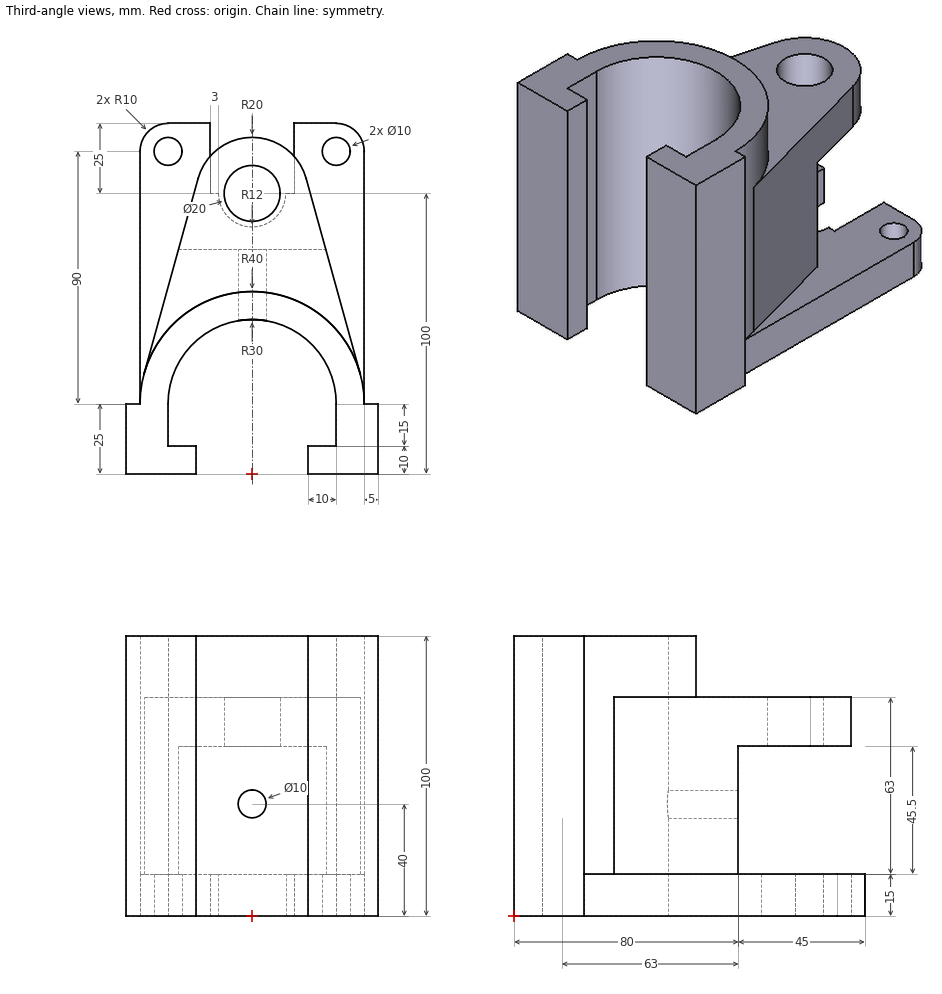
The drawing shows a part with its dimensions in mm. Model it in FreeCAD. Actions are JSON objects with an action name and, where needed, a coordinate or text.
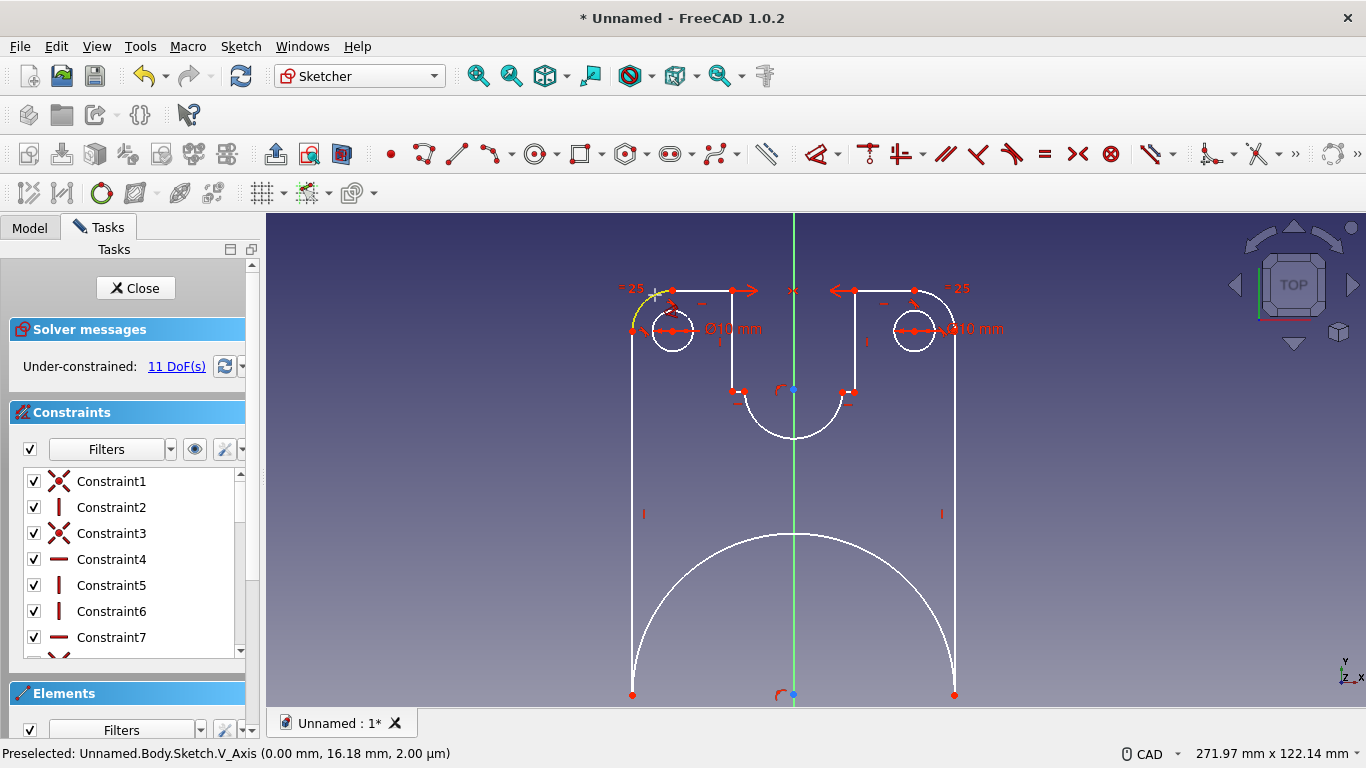
{"action": "left_click", "coordinate": [654, 295]}
{"action": "left_click", "coordinate": [639, 267]}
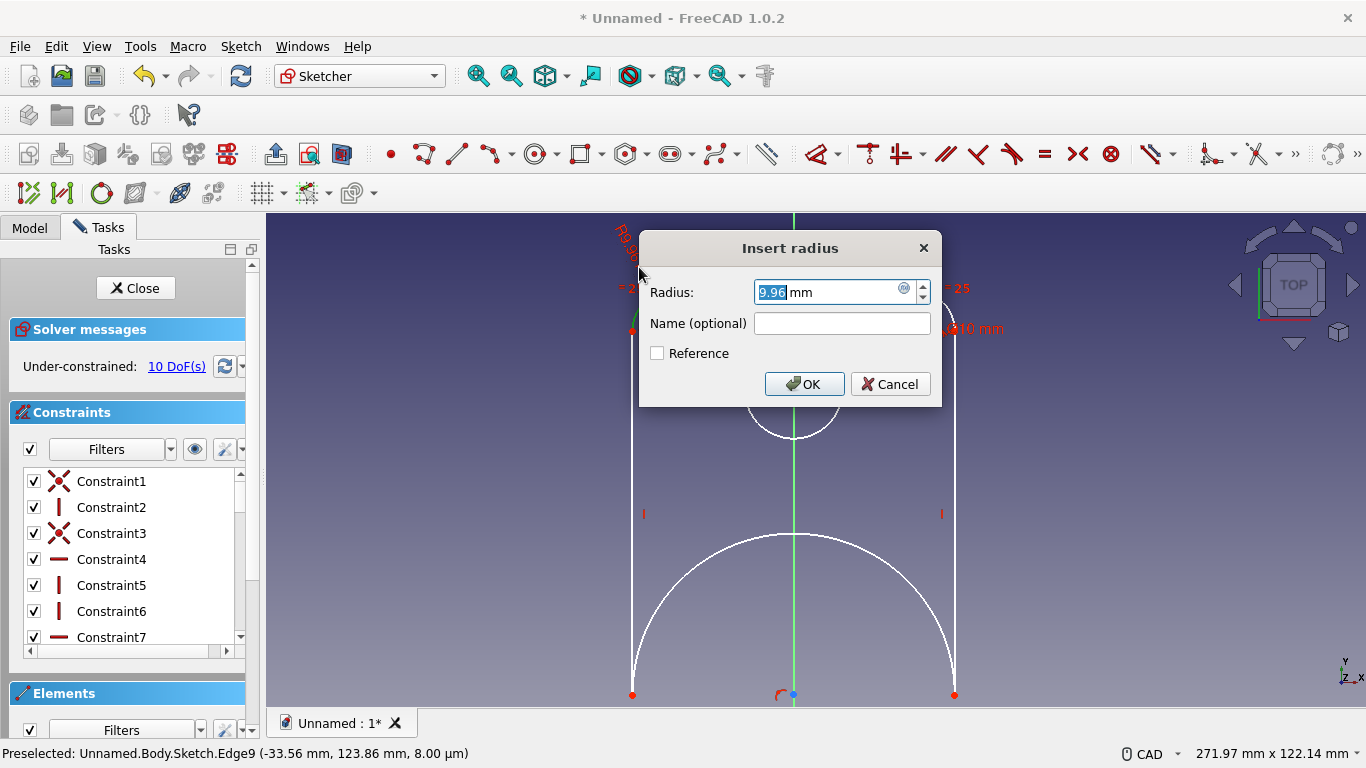
{"action": "type", "text": "10"}
{"action": "key", "text": "Return"}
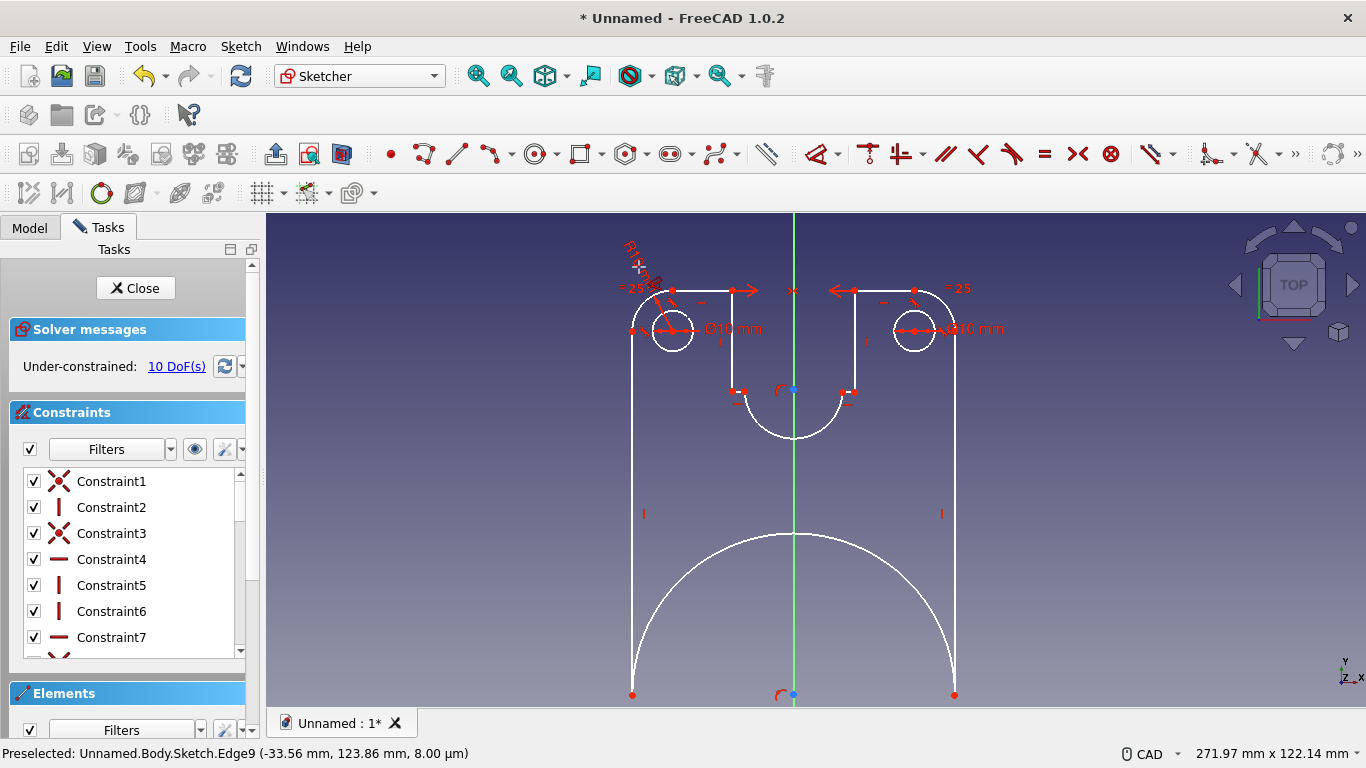
{"action": "left_click", "coordinate": [889, 564]}
{"action": "left_click", "coordinate": [908, 538]}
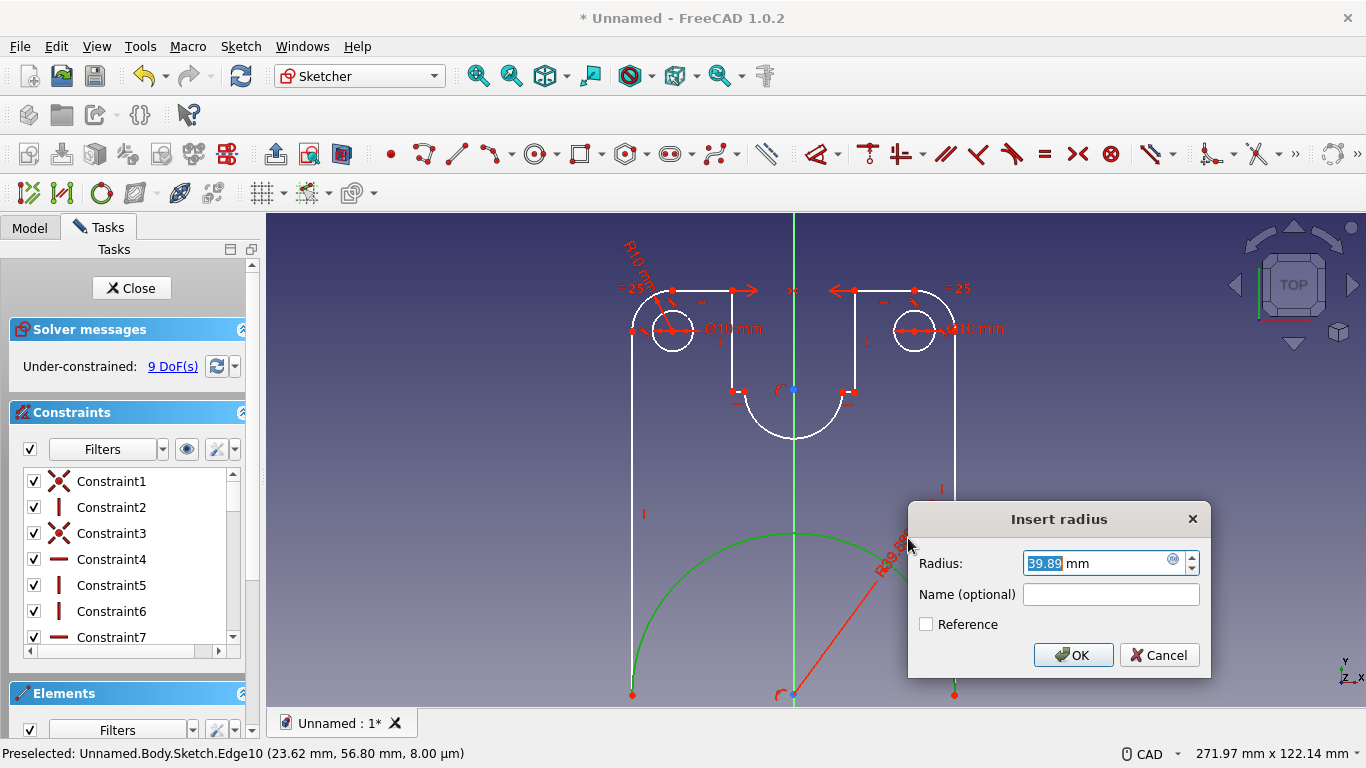
{"action": "type", "text": "40"}
{"action": "key", "text": "Return"}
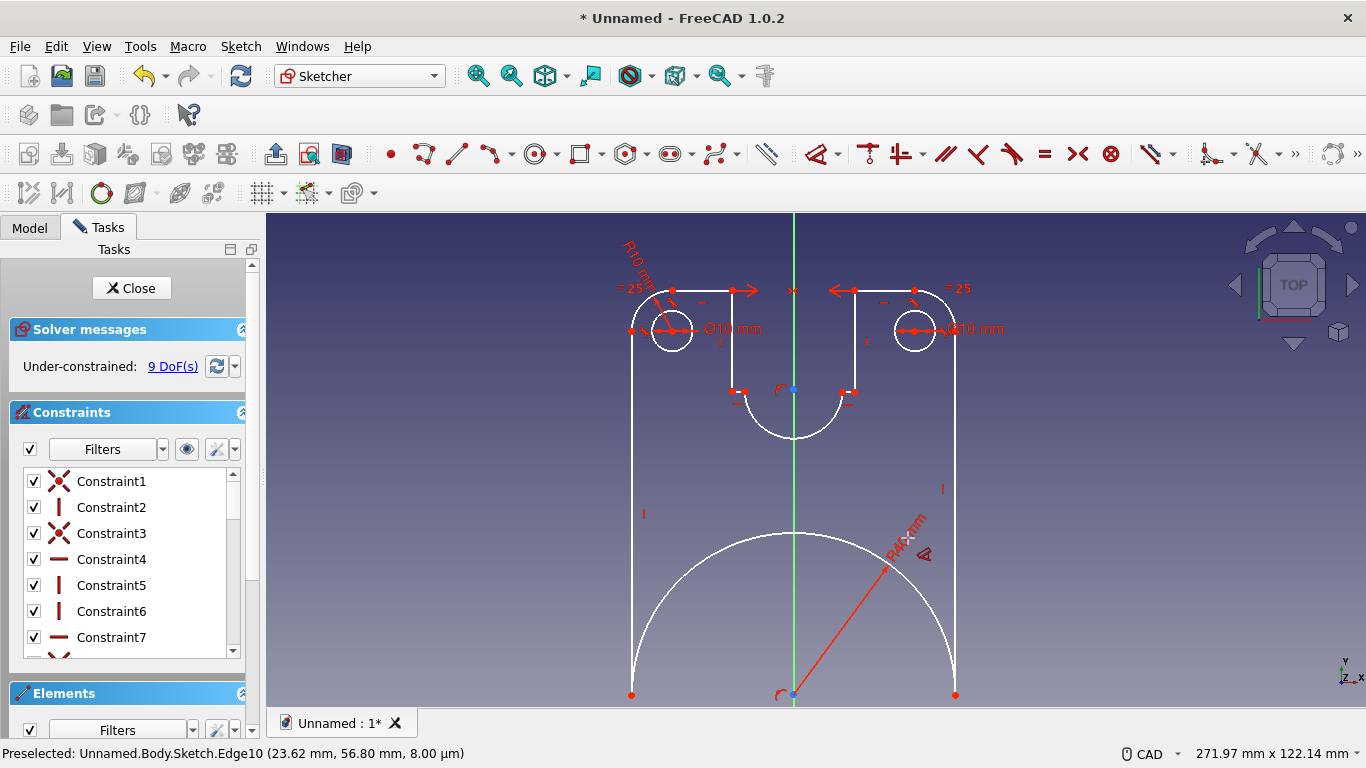
{"action": "left_click", "coordinate": [765, 430]}
{"action": "left_click", "coordinate": [746, 456]}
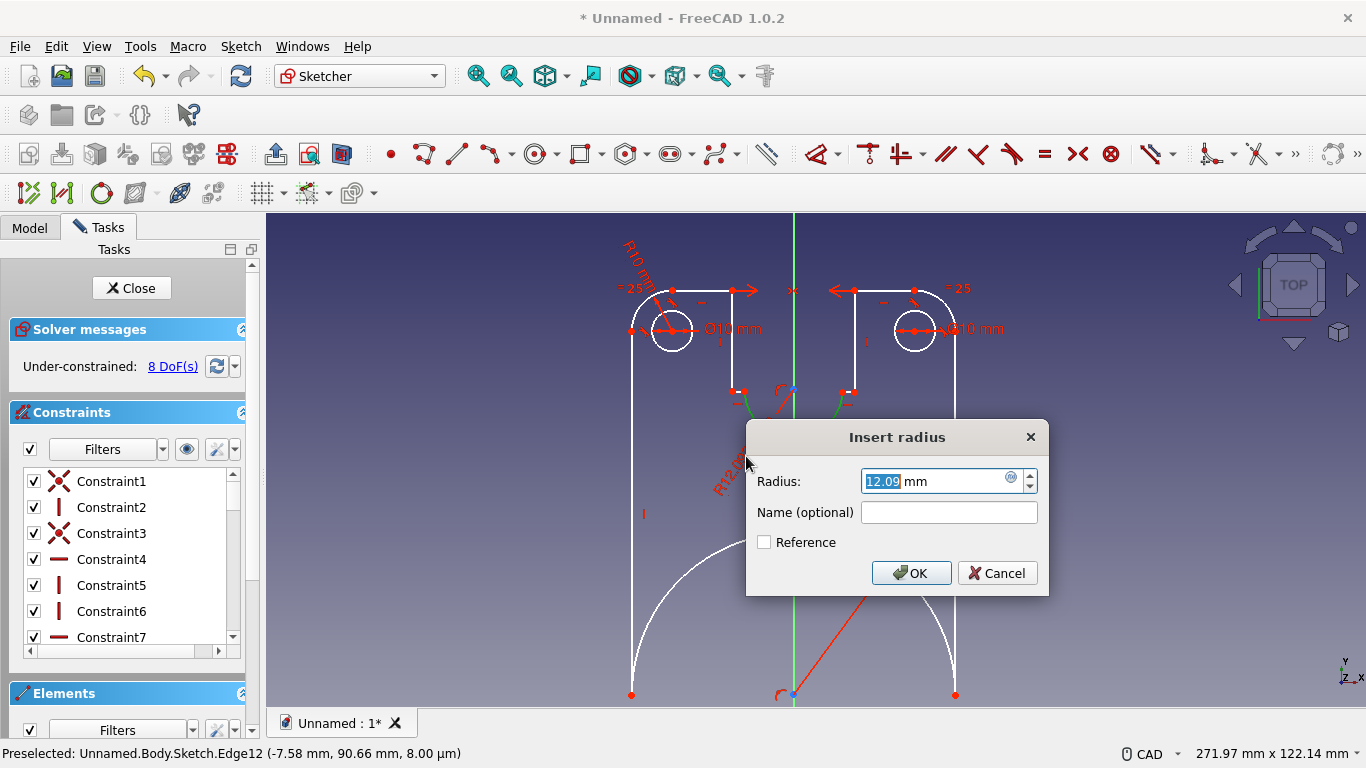
{"action": "type", "text": "12"}
{"action": "key", "text": "Return"}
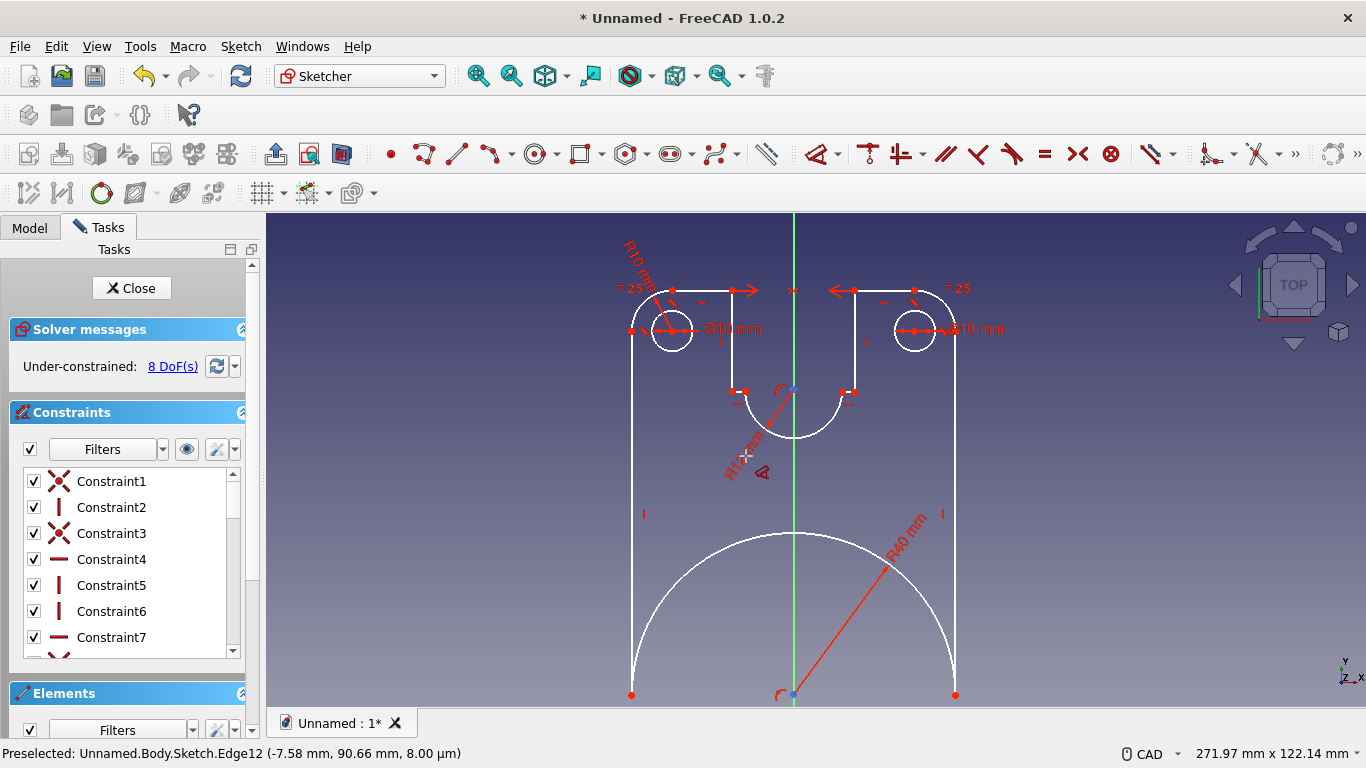
{"action": "scroll", "coordinate": [739, 392], "scroll_direction": "up", "scroll_amount": 6}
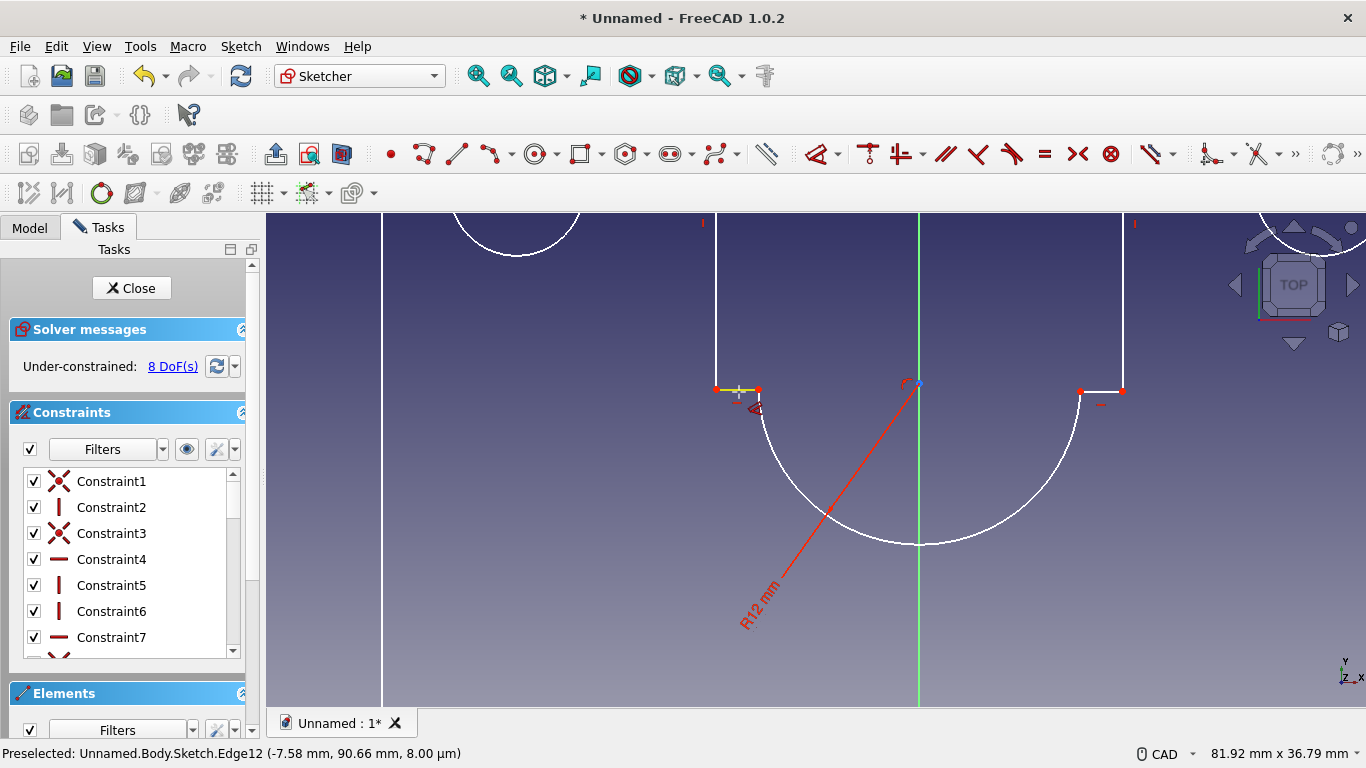
{"action": "left_click", "coordinate": [737, 390]}
{"action": "left_click", "coordinate": [737, 356]}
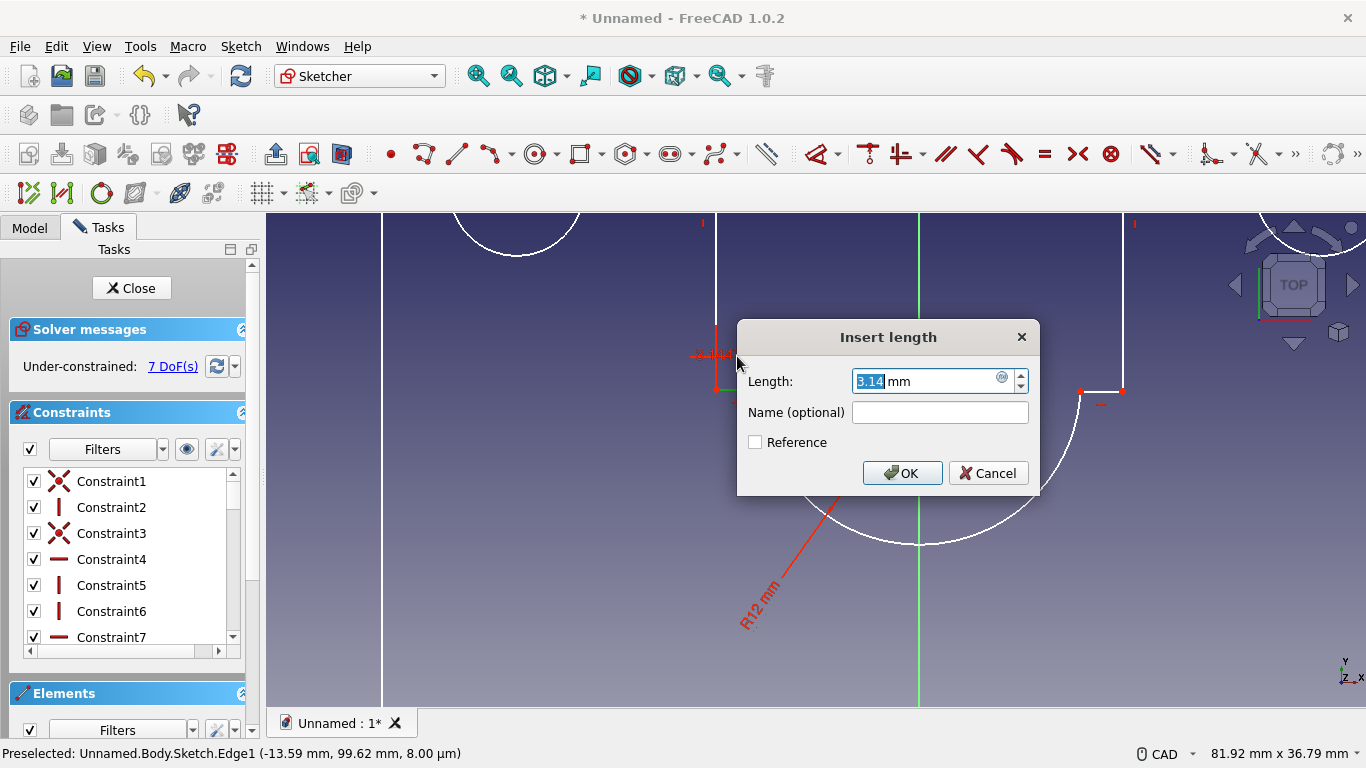
{"action": "type", "text": "3"}
{"action": "key", "text": "Return"}